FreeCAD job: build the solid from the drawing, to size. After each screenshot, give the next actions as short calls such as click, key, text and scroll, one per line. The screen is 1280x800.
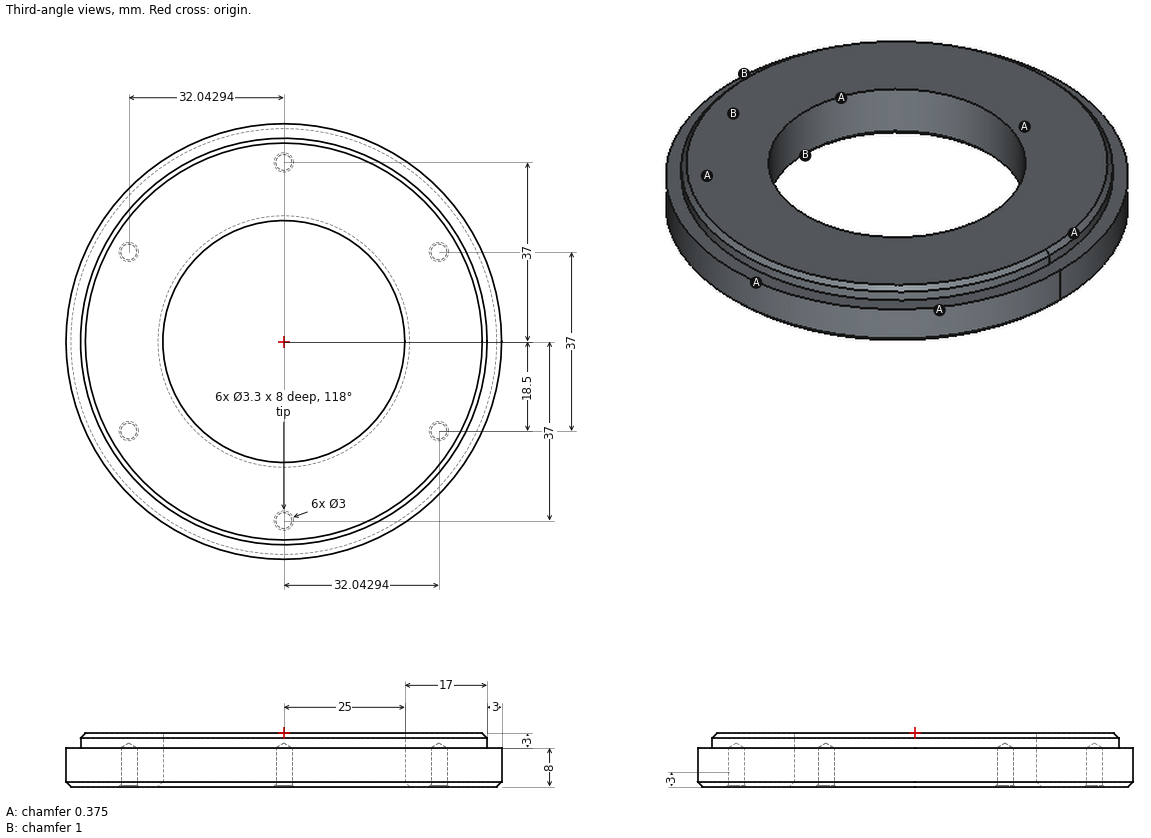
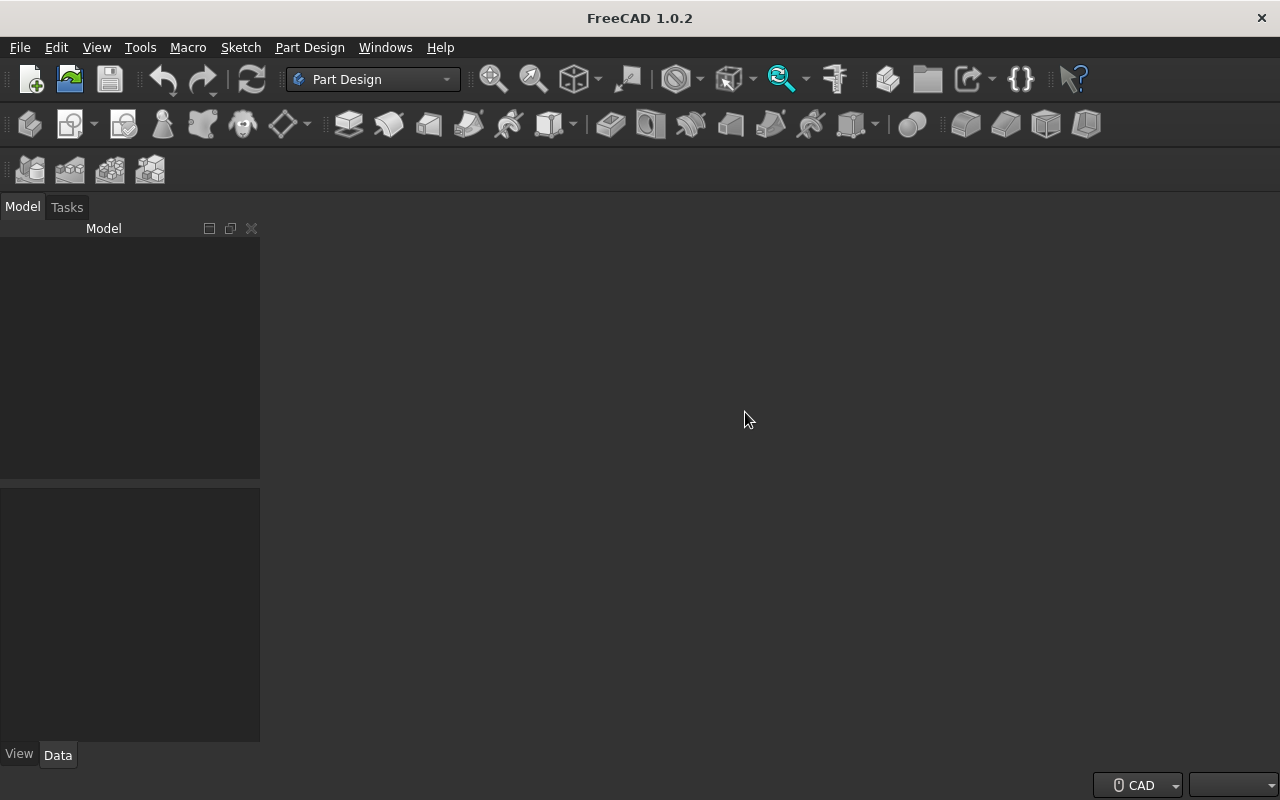
click(30, 80)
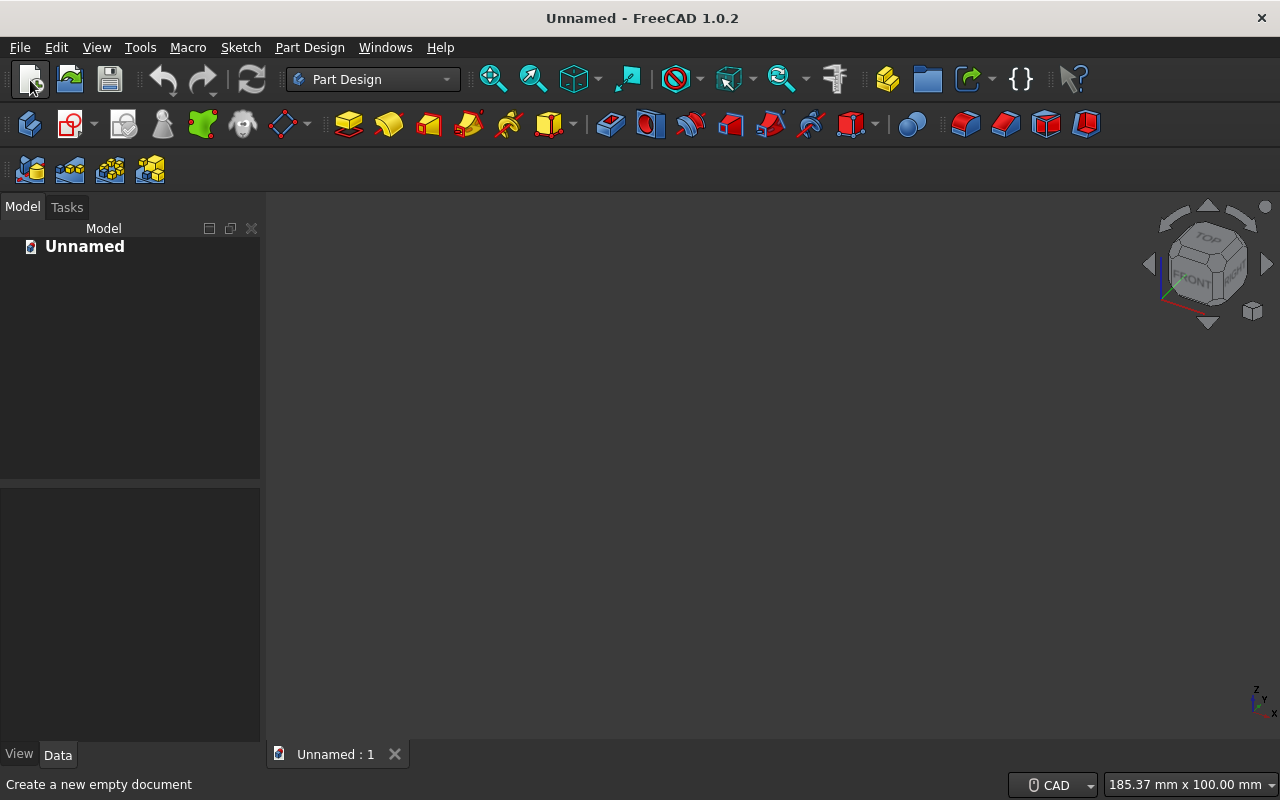
click(70, 124)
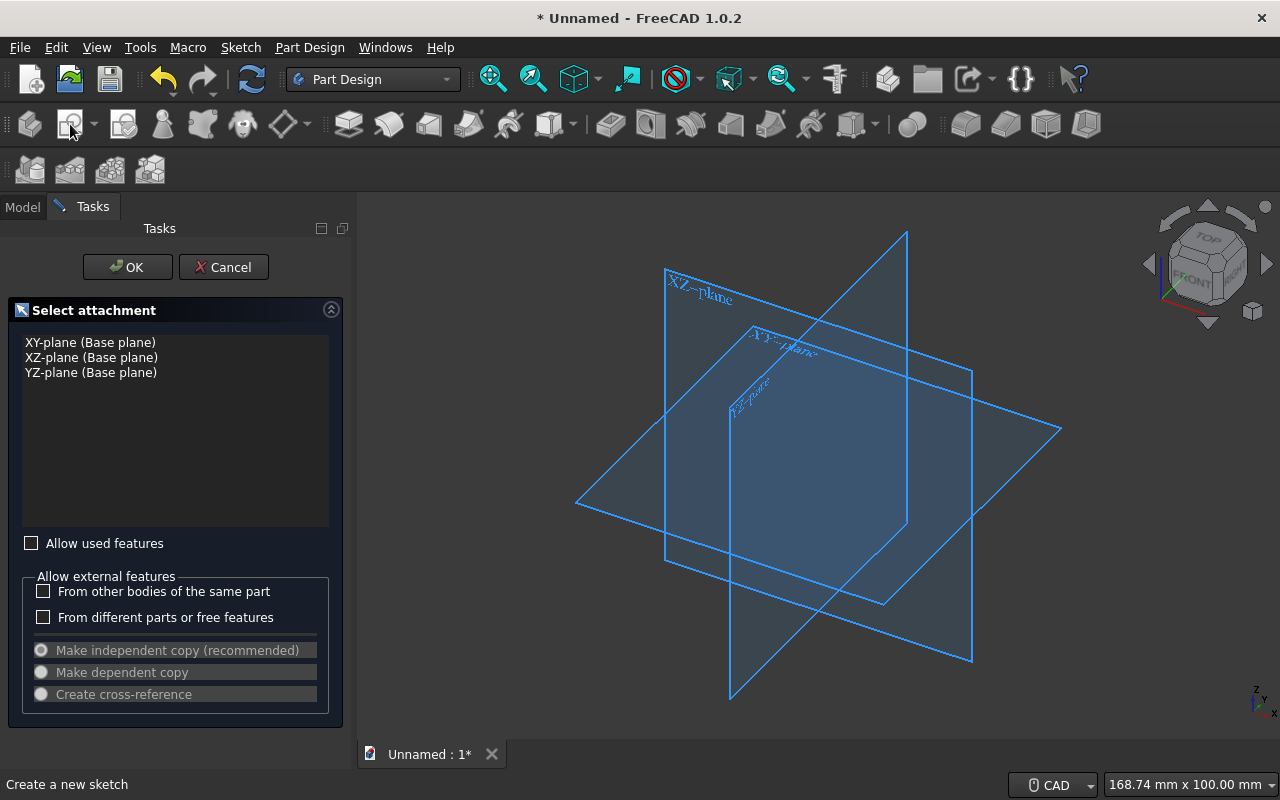
click(82, 358)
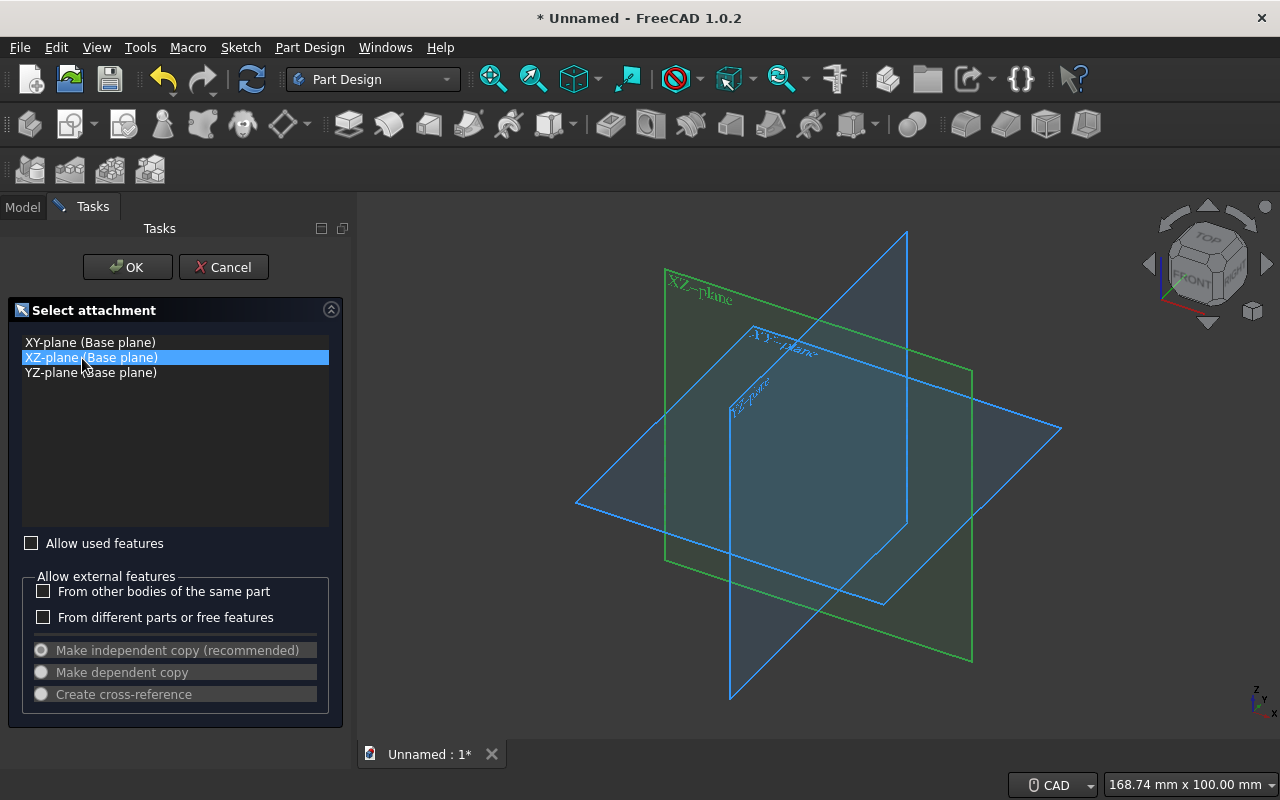
click(128, 267)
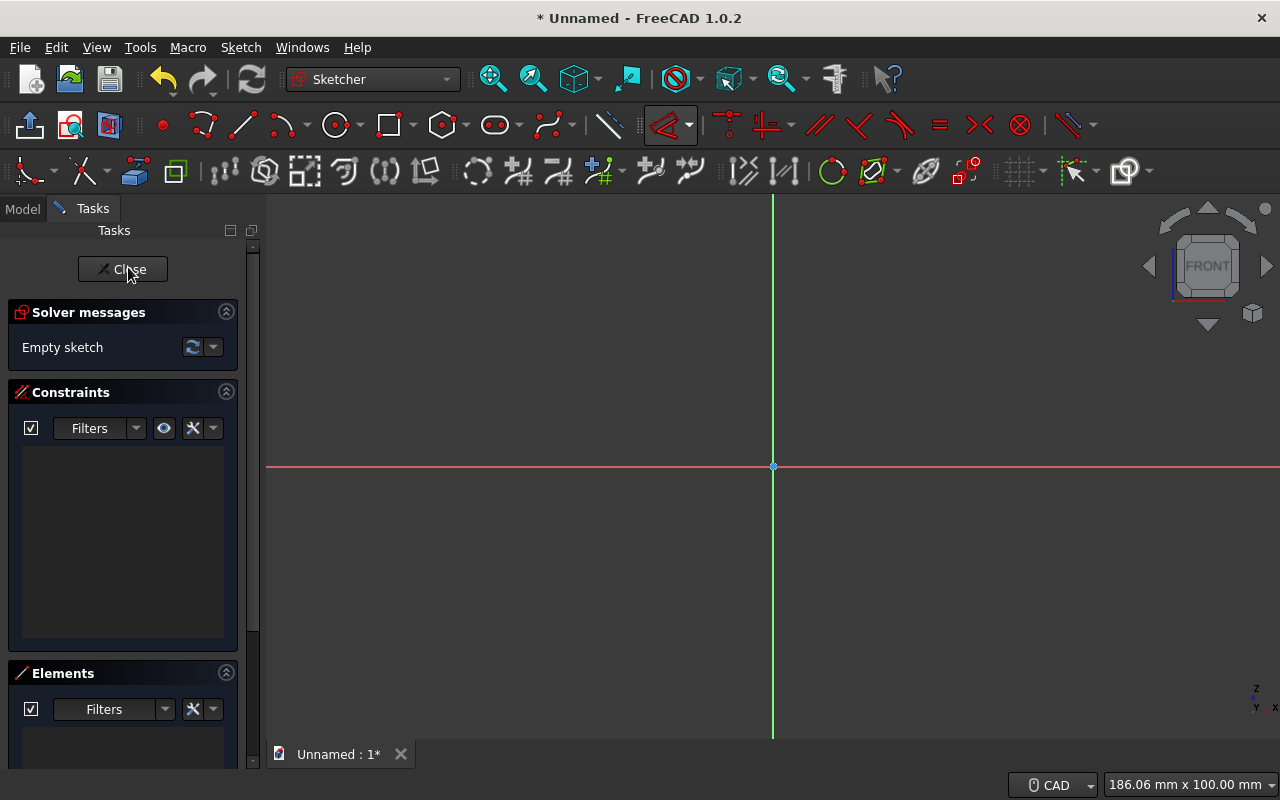
scroll(1052, 521, up, 4)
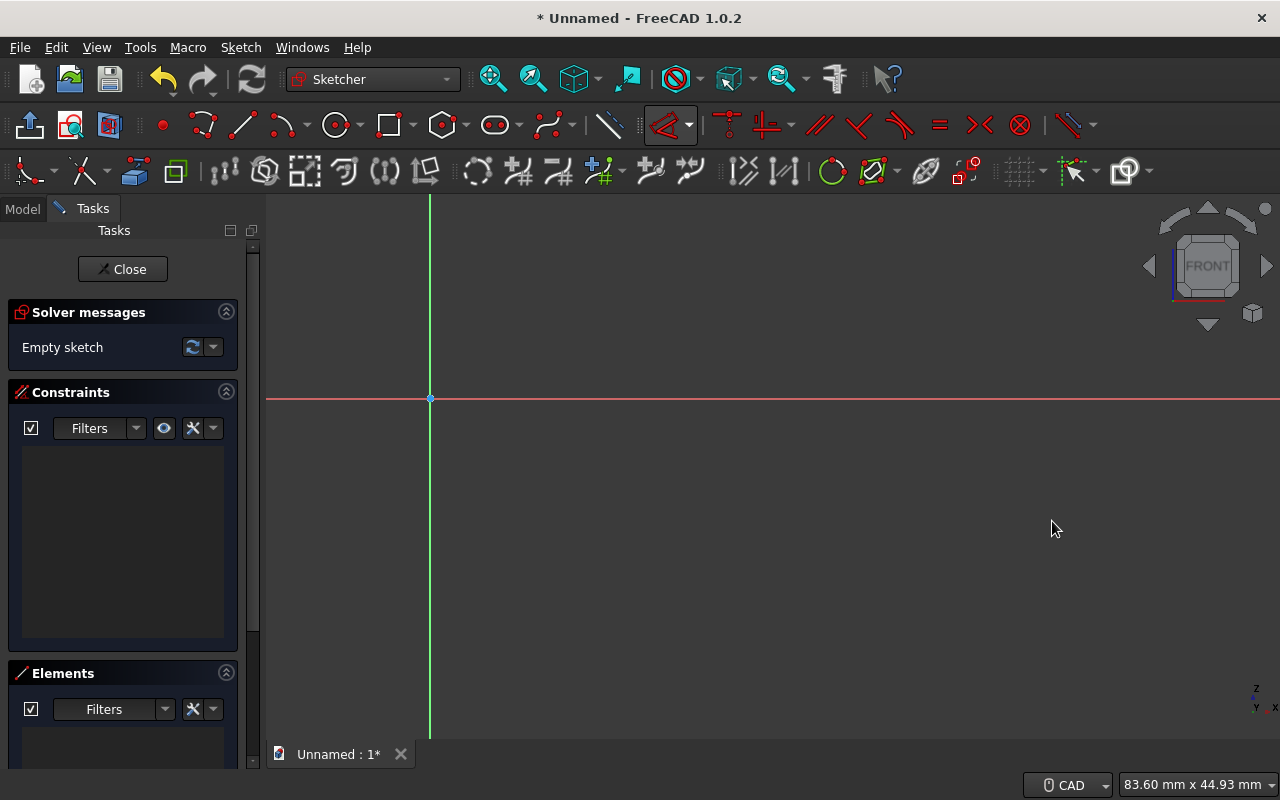
click(204, 126)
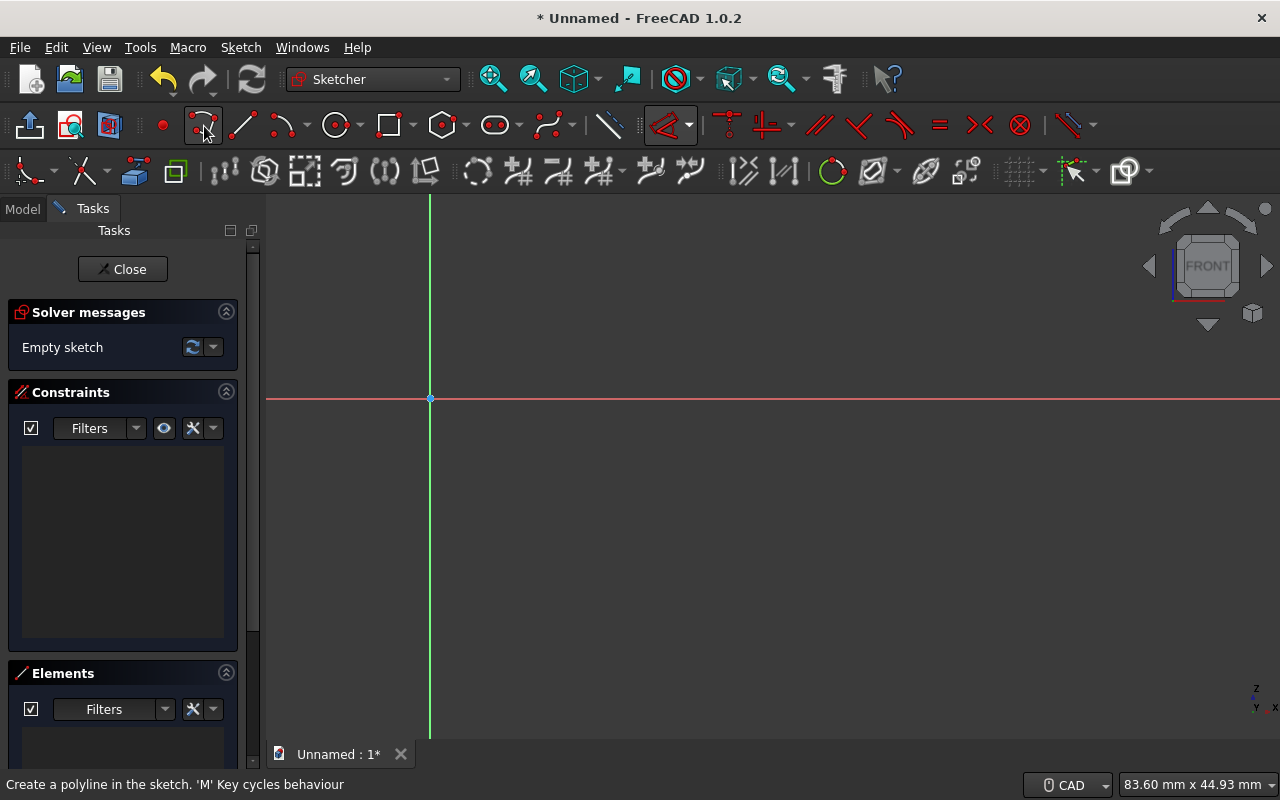
click(733, 399)
click(940, 408)
click(940, 435)
click(976, 435)
click(976, 532)
click(733, 532)
click(733, 399)
key(Escape)
key(Escape)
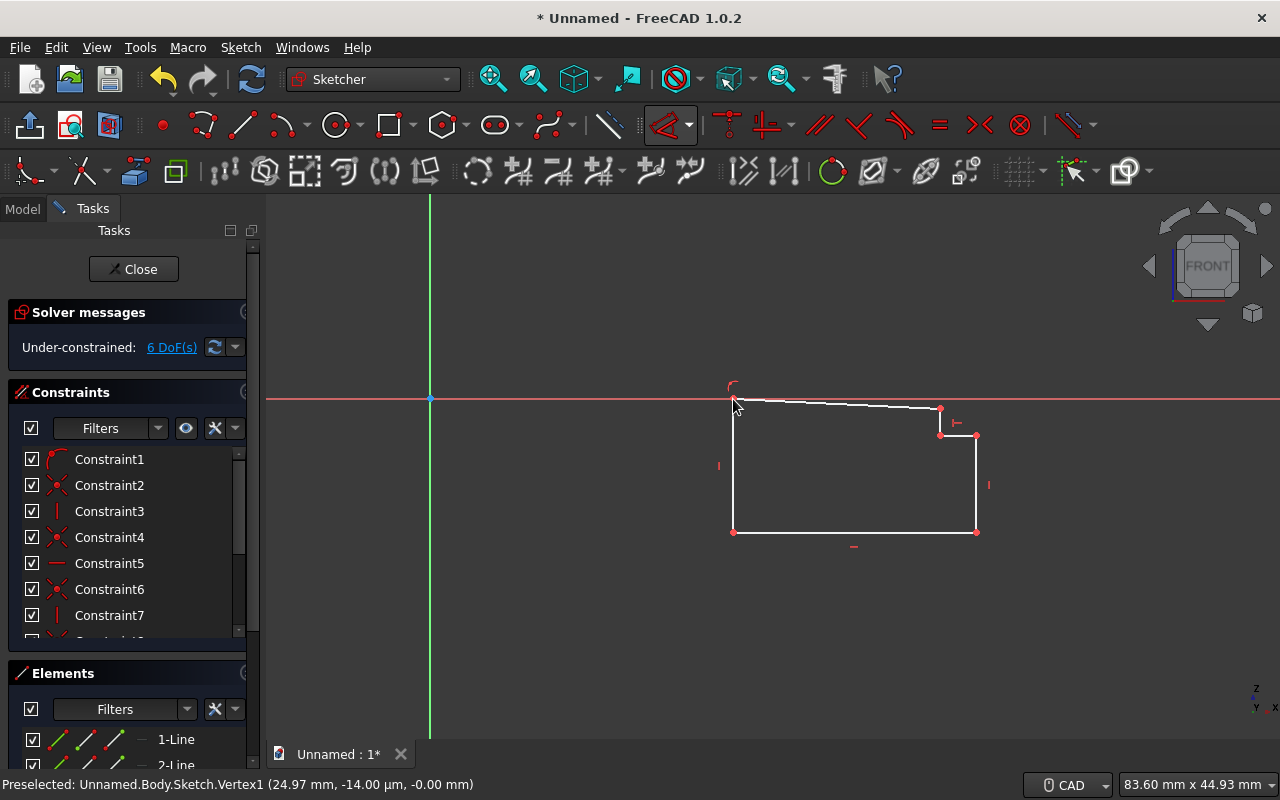
click(795, 402)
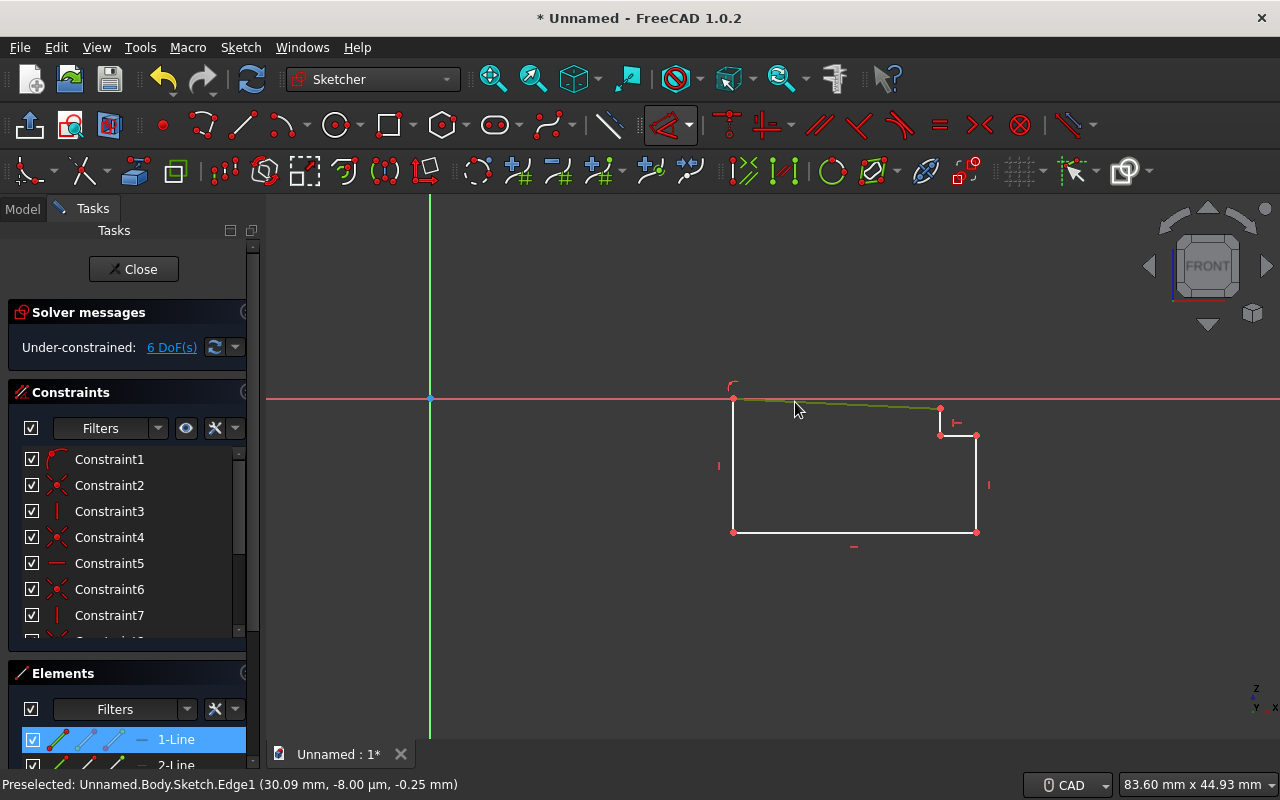
click(794, 126)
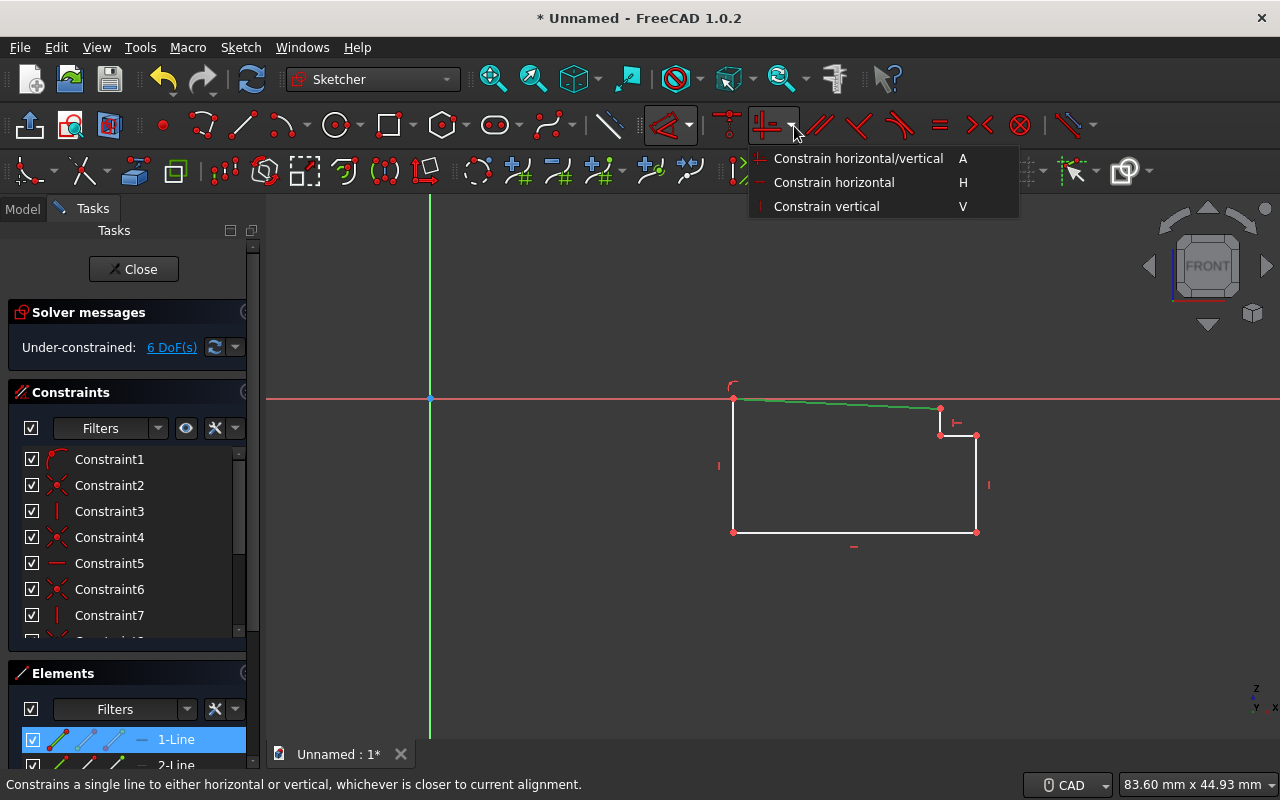
click(884, 182)